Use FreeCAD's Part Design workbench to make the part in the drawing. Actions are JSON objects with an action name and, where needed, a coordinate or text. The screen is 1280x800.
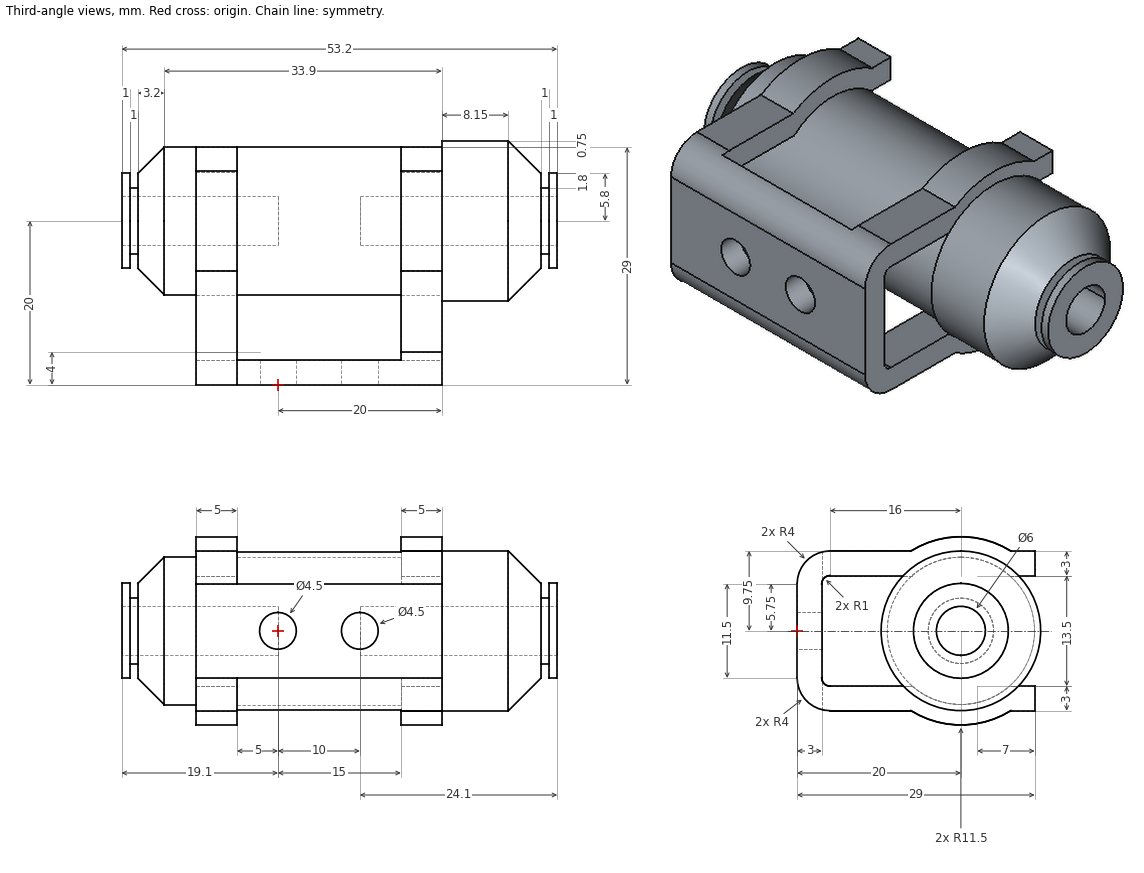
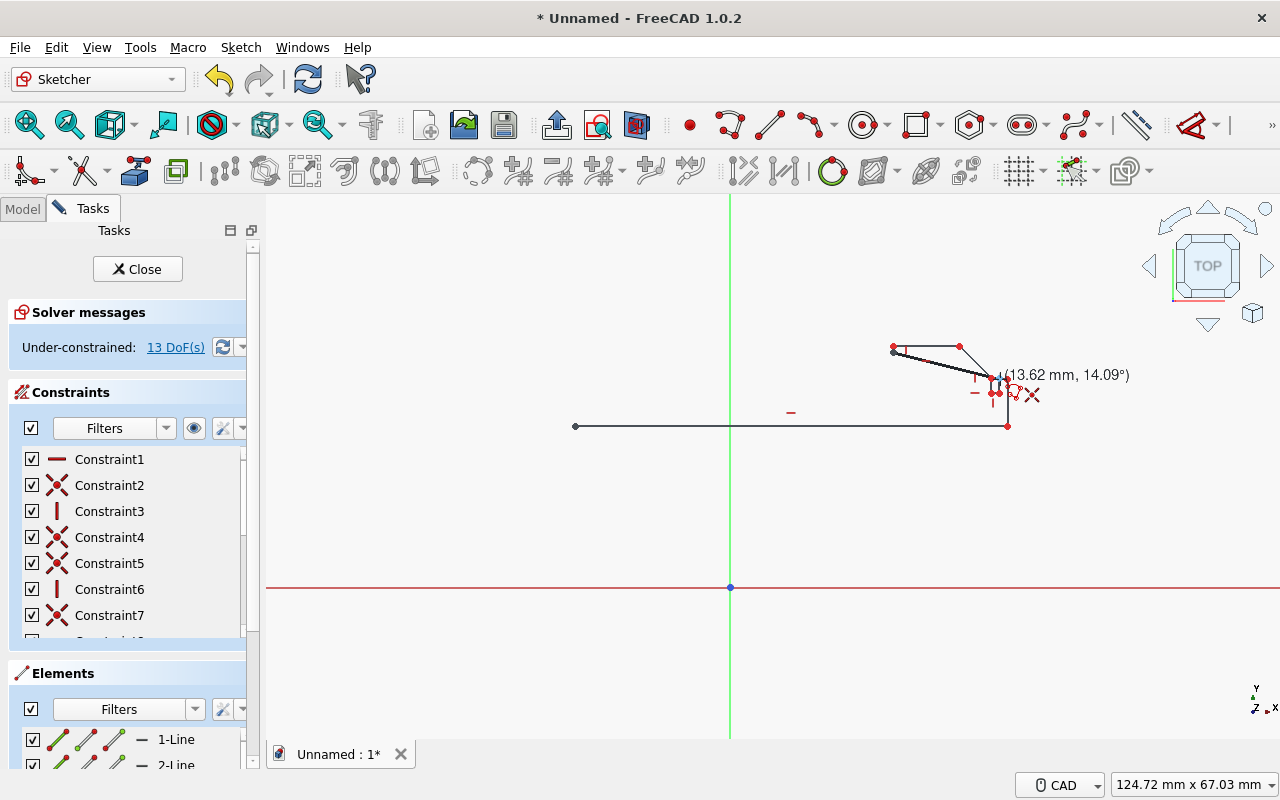
{"action": "left_click", "coordinate": [617, 352]}
{"action": "left_click", "coordinate": [591, 378]}
{"action": "left_click", "coordinate": [591, 393]}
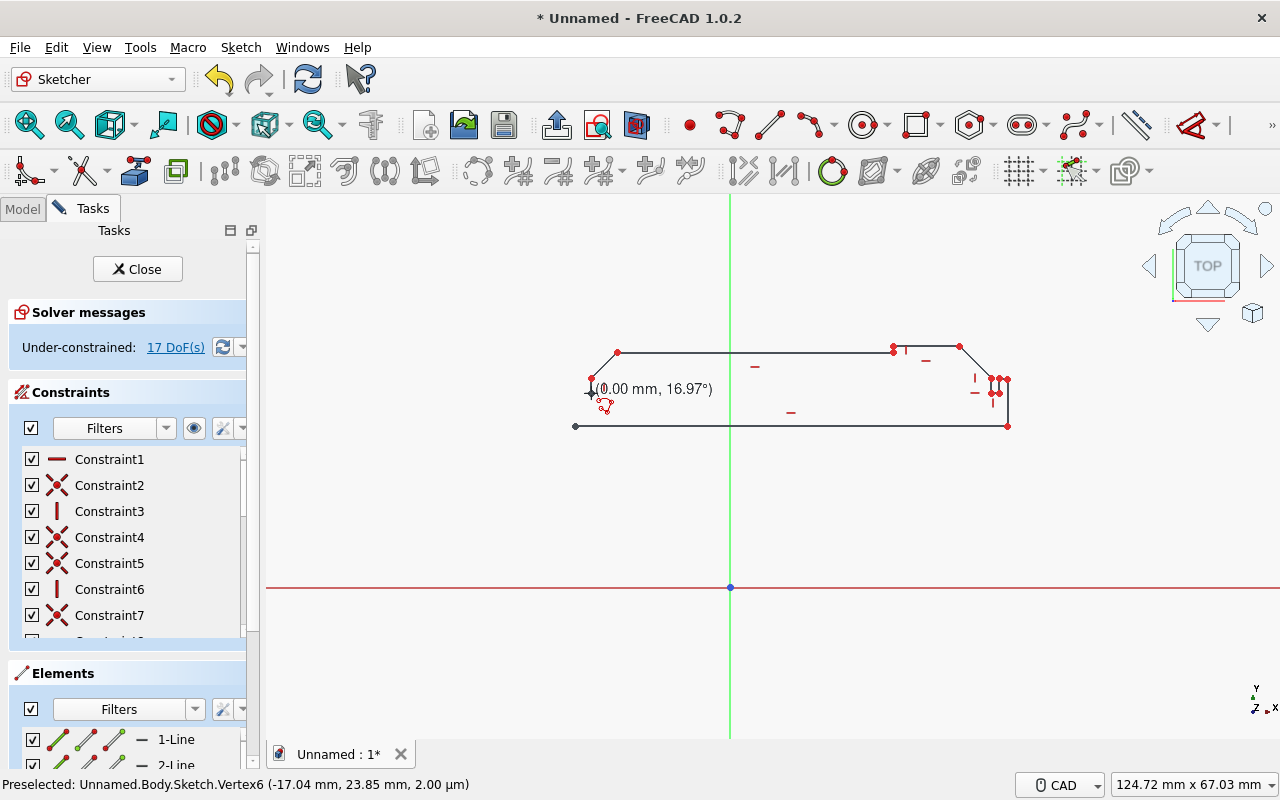
{"action": "scroll", "coordinate": [583, 393], "scroll_direction": "up", "scroll_amount": 4}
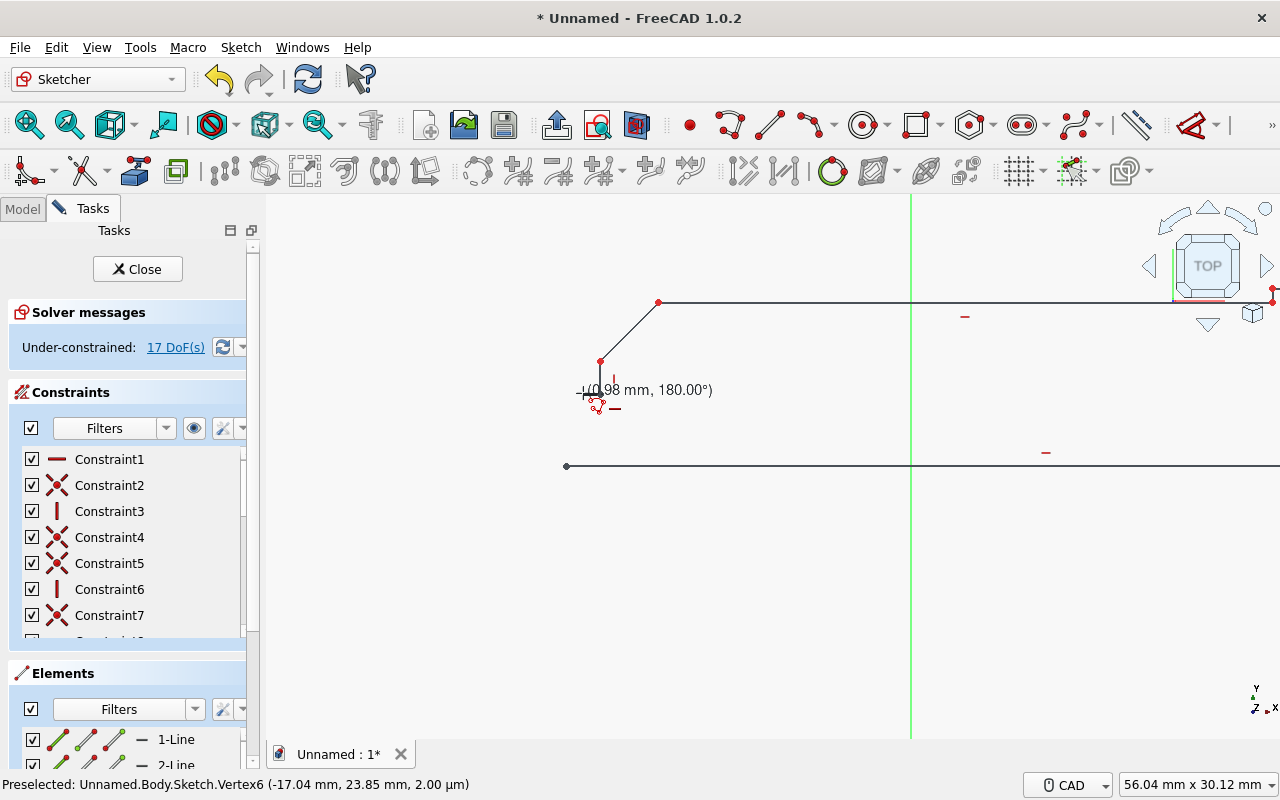
{"action": "left_click", "coordinate": [583, 393]}
{"action": "left_click", "coordinate": [583, 359]}
{"action": "left_click", "coordinate": [565, 359]}
{"action": "left_click", "coordinate": [566, 466]}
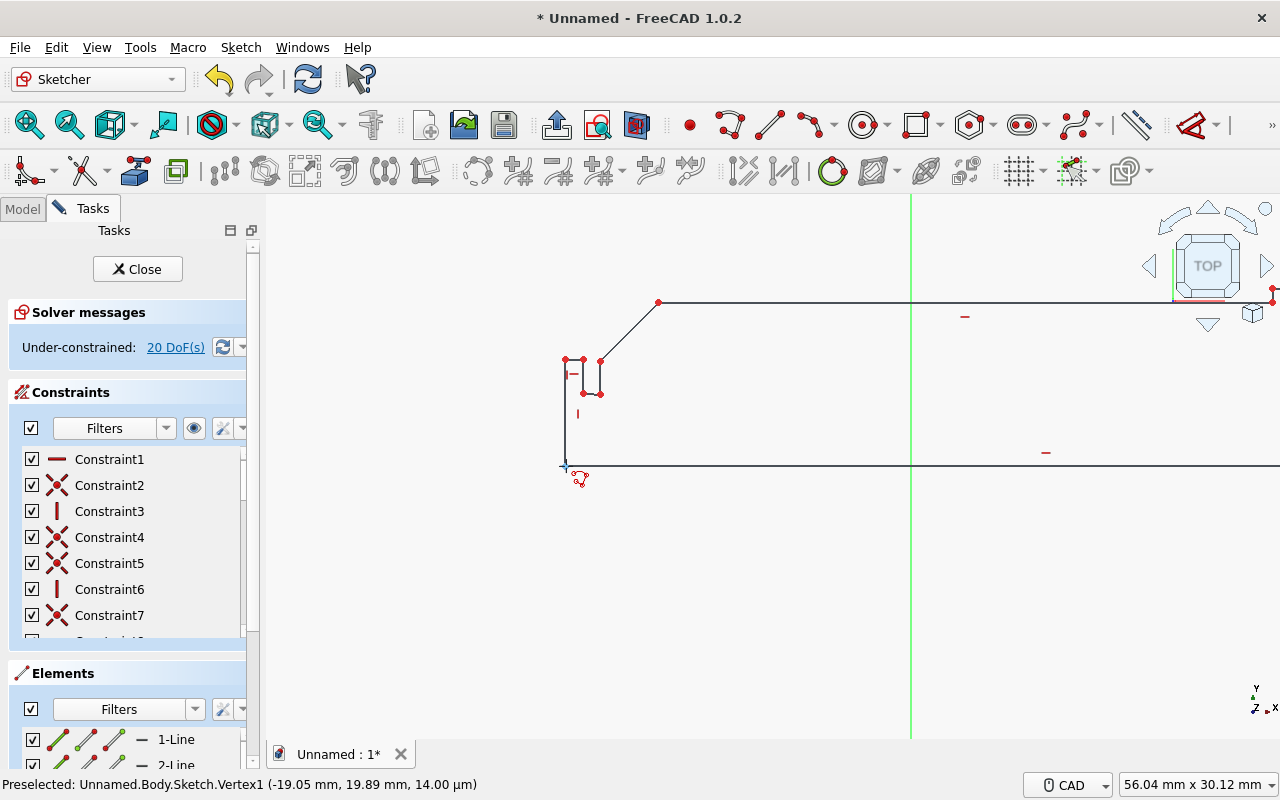
{"action": "left_click", "coordinate": [770, 126]}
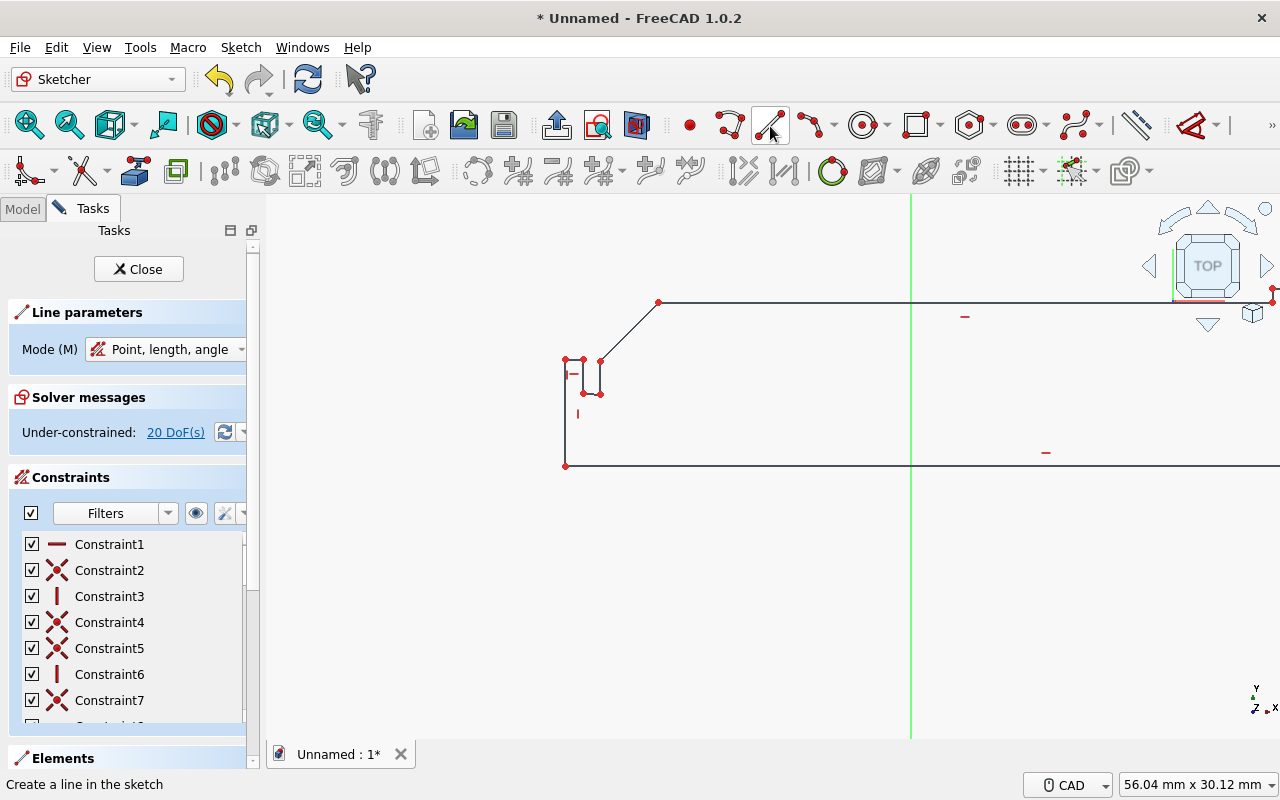
{"action": "left_click", "coordinate": [469, 464]}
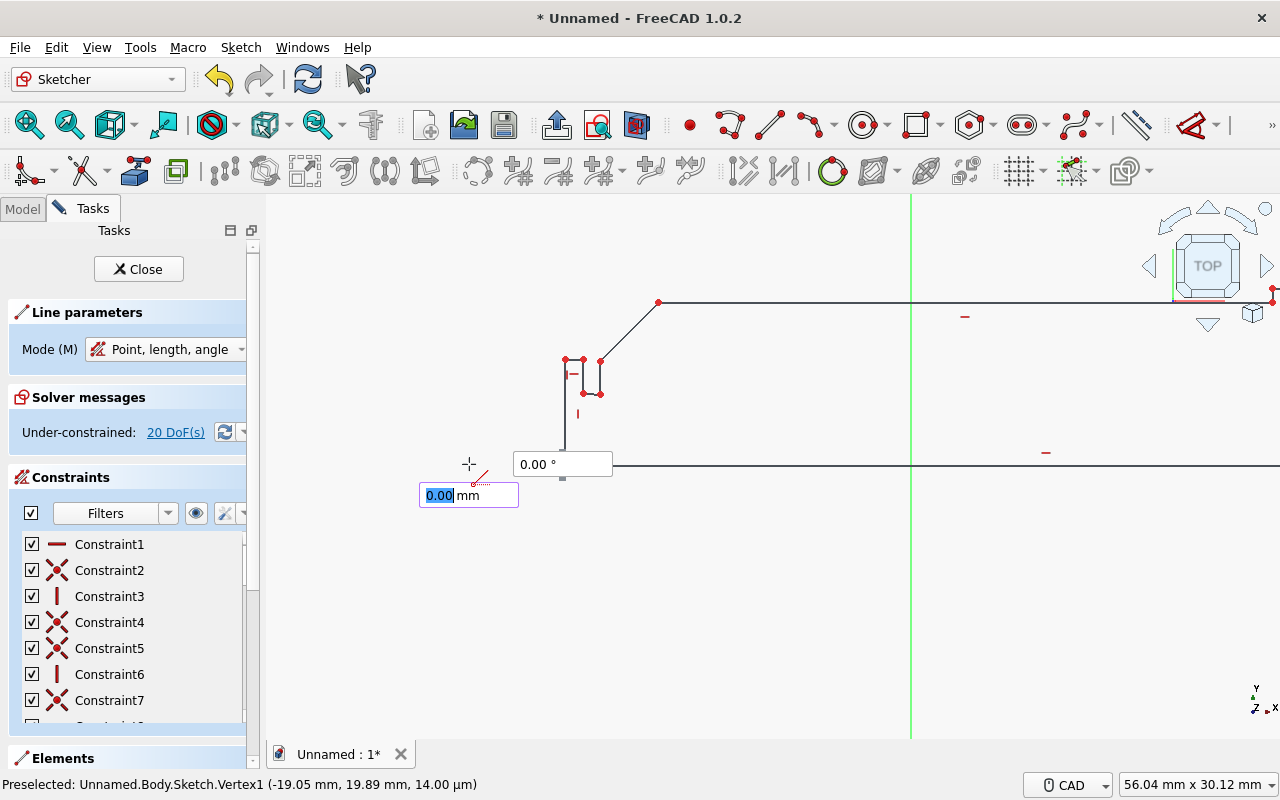
{"action": "scroll", "coordinate": [583, 393], "scroll_direction": "down", "scroll_amount": 4}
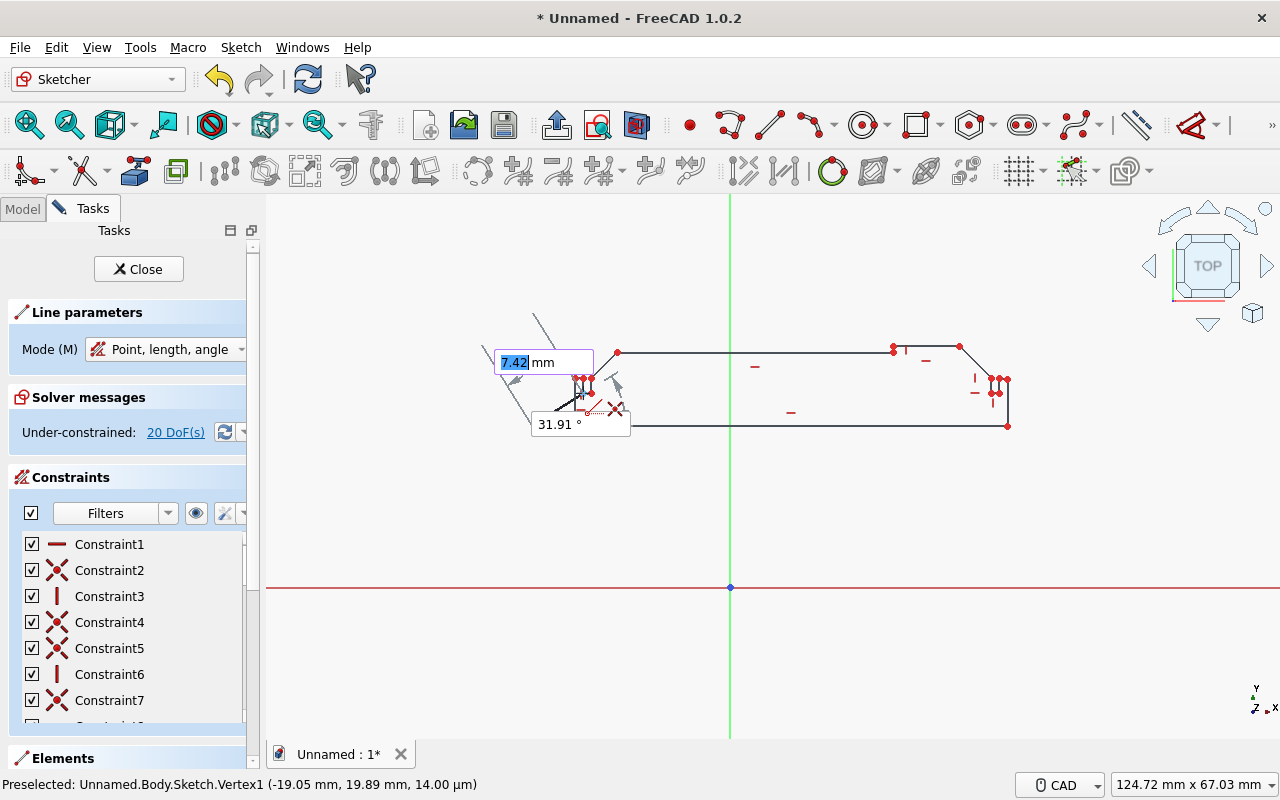
{"action": "left_click", "coordinate": [402, 425]}
{"action": "key", "text": "Escape"}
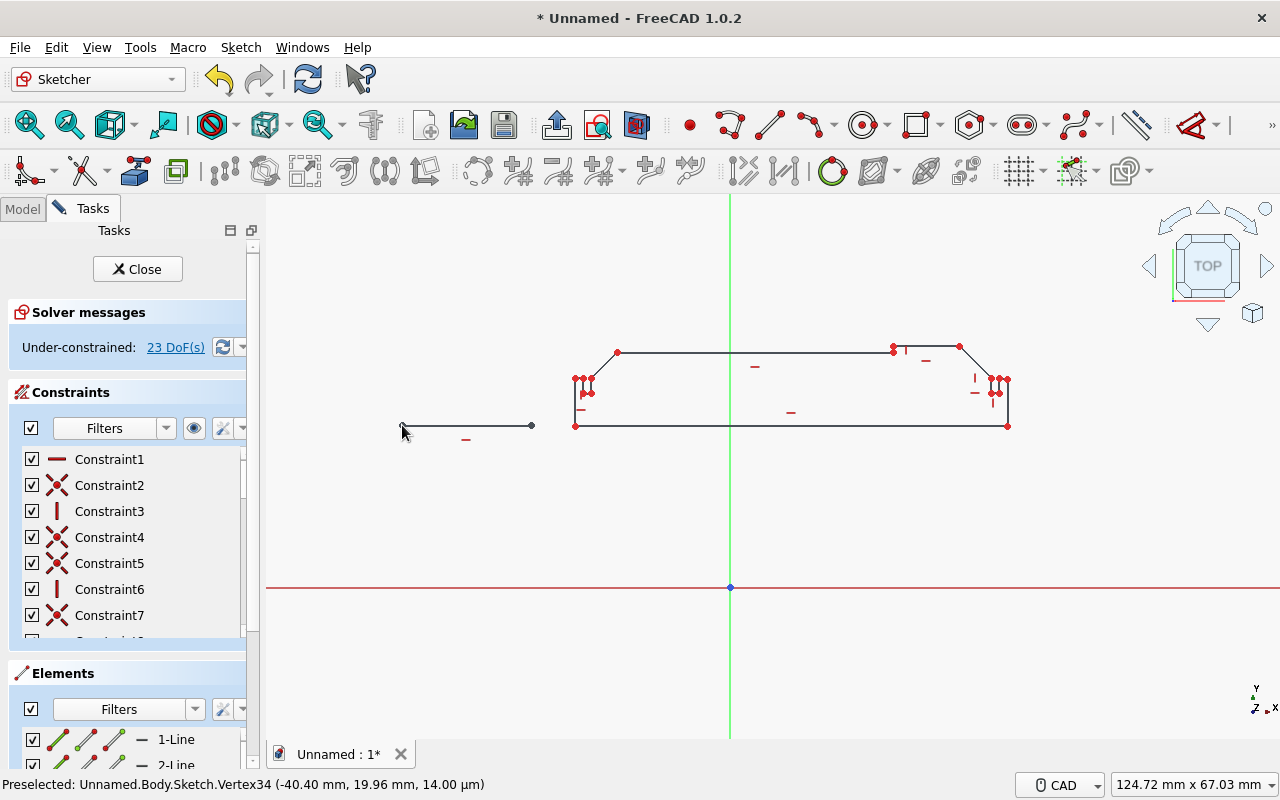
{"action": "left_click", "coordinate": [493, 426]}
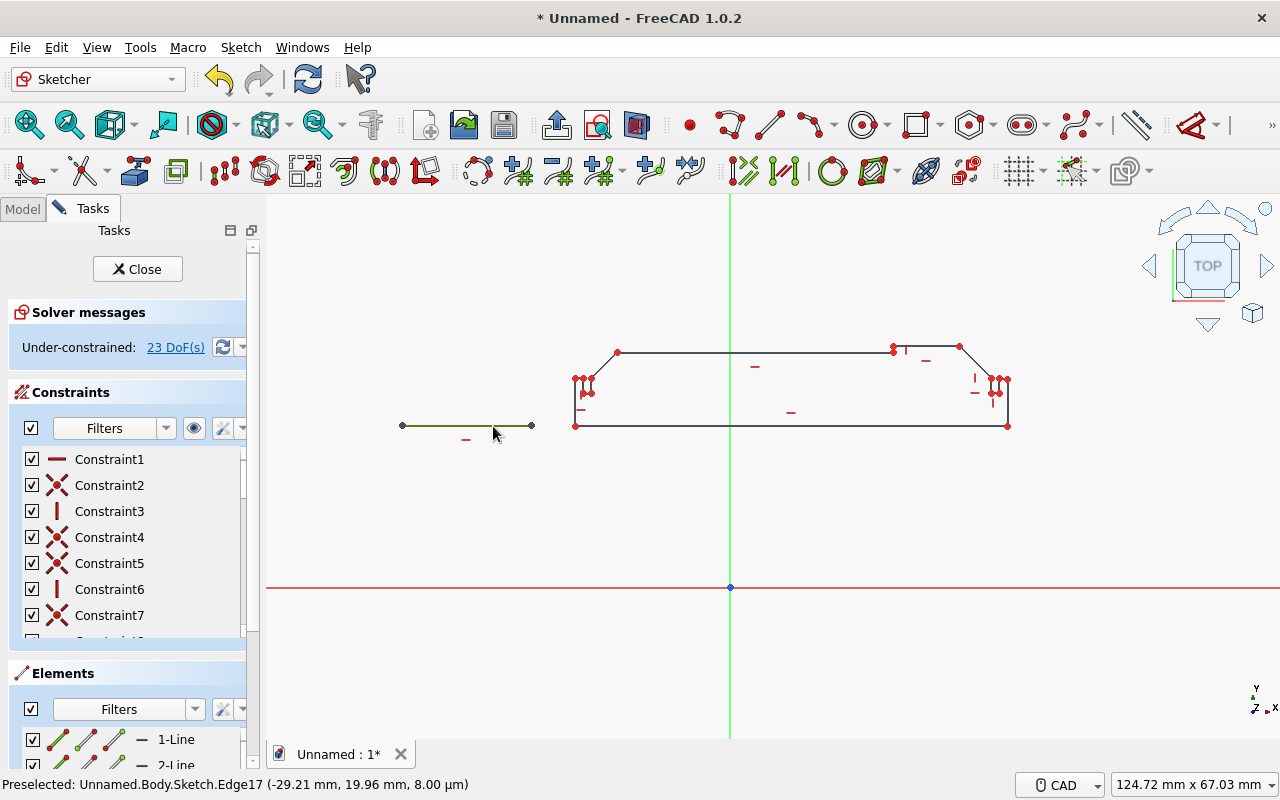
{"action": "left_click", "coordinate": [1138, 126]}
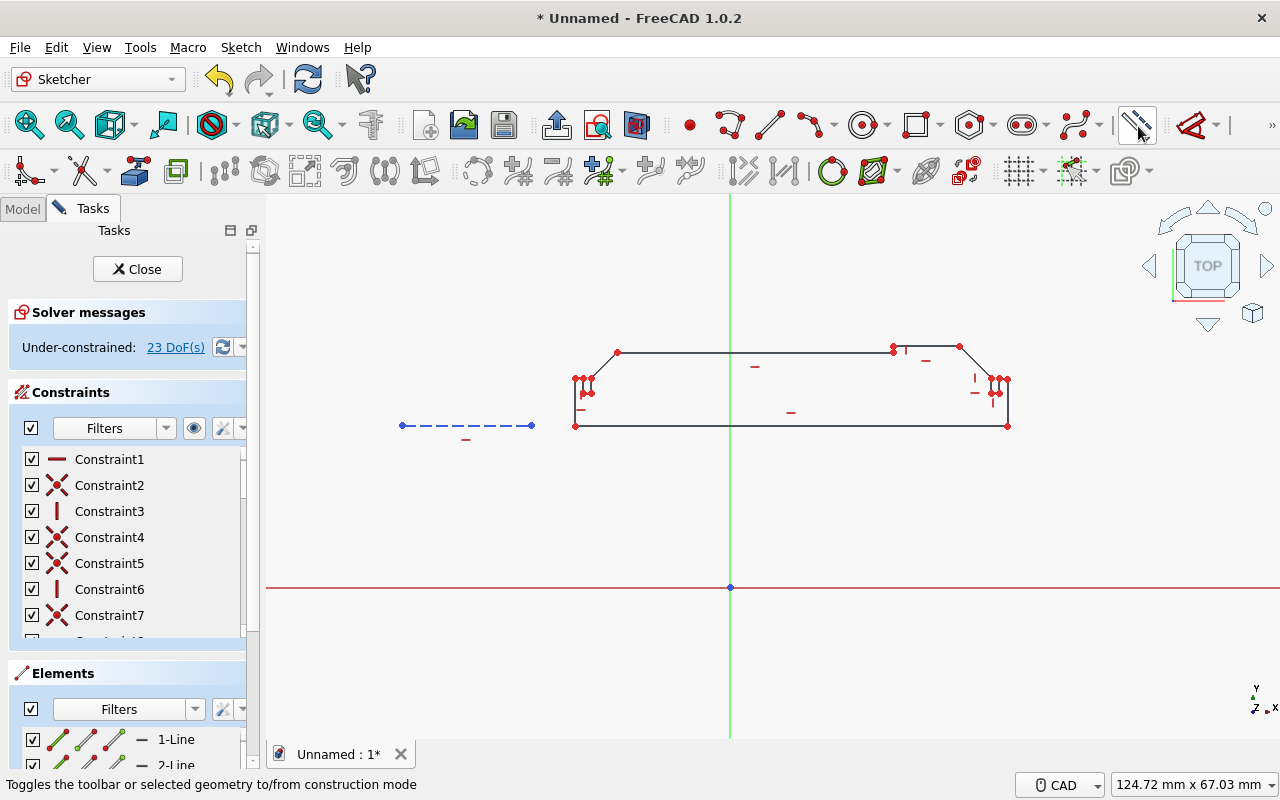
{"action": "scroll", "coordinate": [1004, 379], "scroll_direction": "up", "scroll_amount": 7}